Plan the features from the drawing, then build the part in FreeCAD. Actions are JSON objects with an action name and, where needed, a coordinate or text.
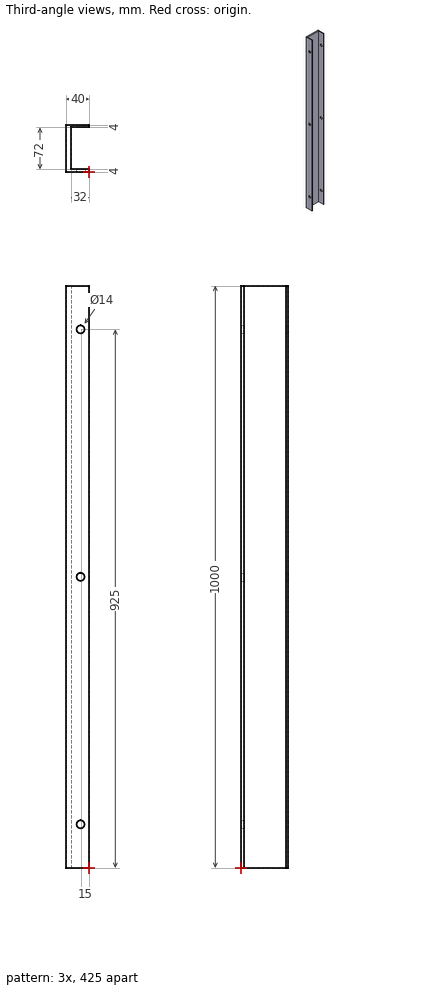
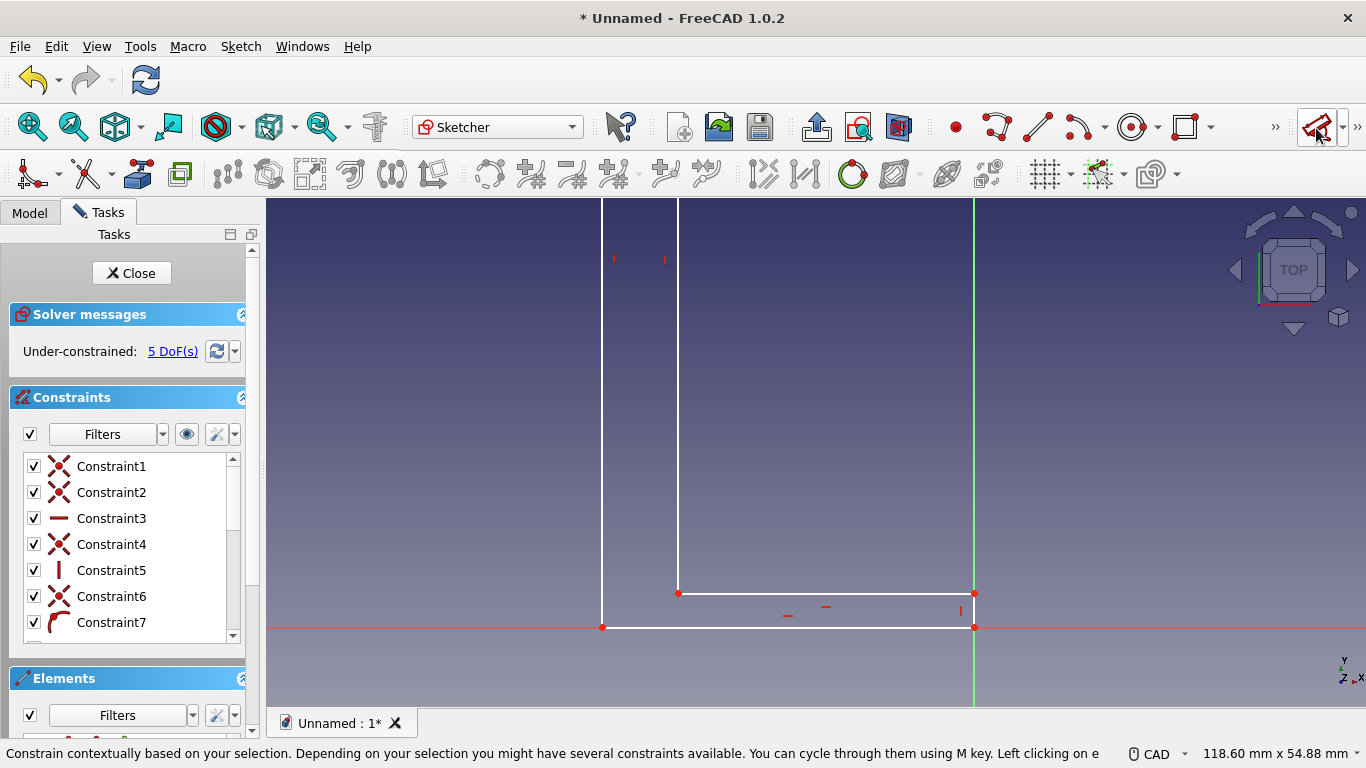
{"action": "scroll", "coordinate": [974, 618], "scroll_direction": "up", "scroll_amount": 2}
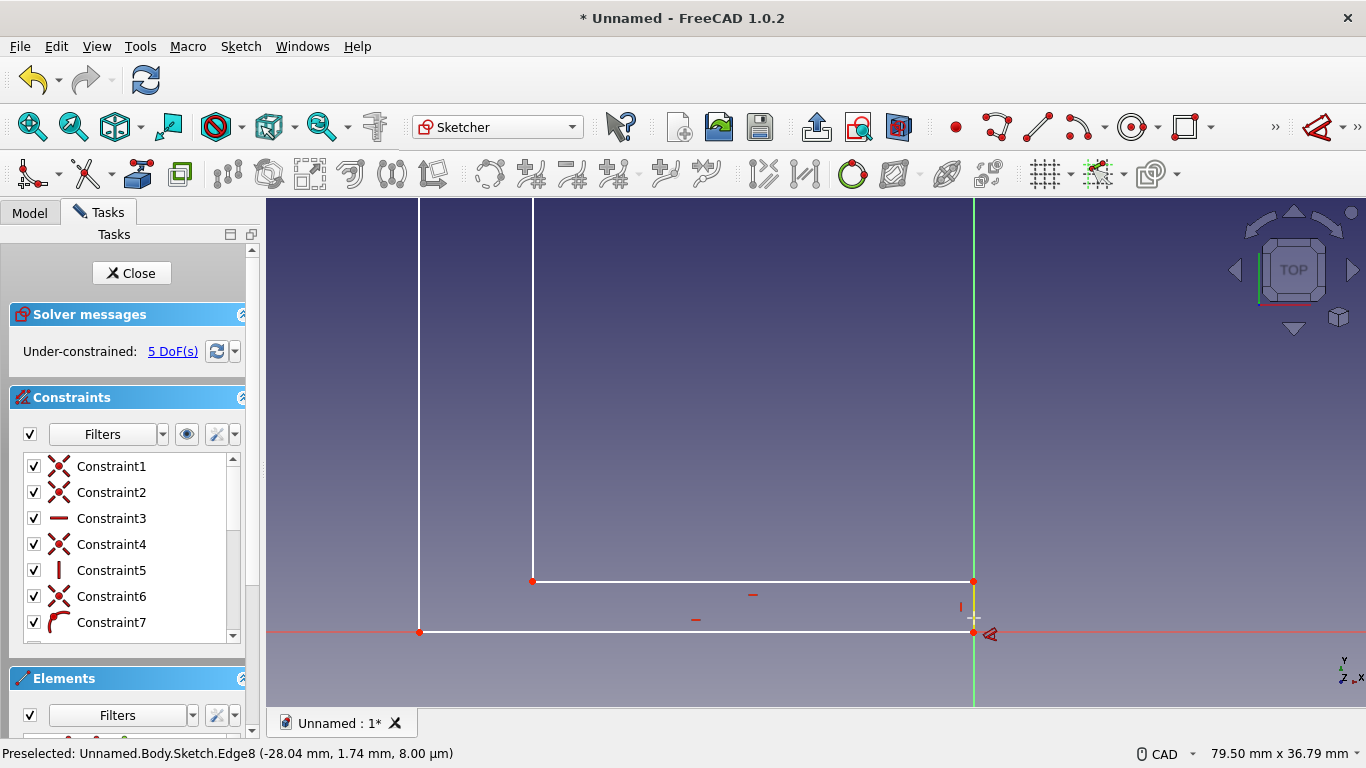
{"action": "left_click", "coordinate": [974, 617]}
{"action": "left_click", "coordinate": [1008, 607]}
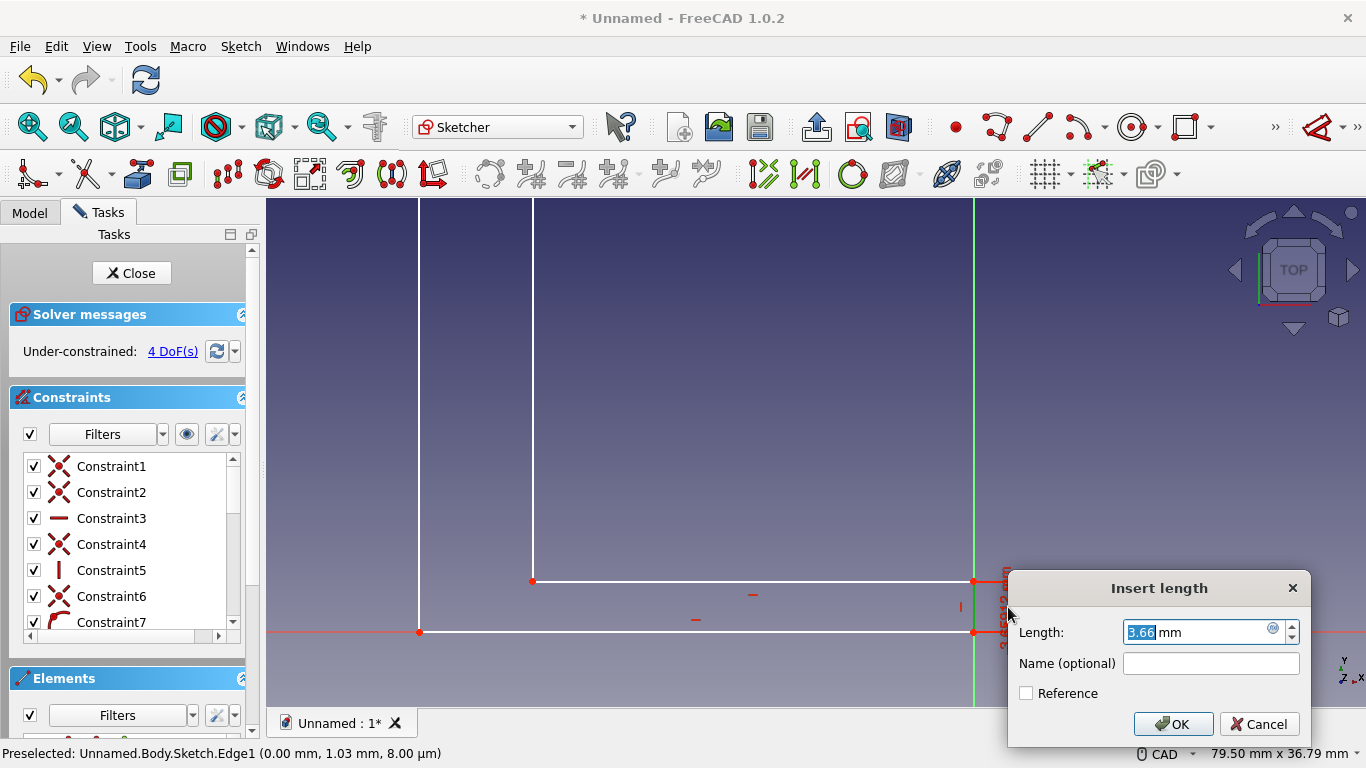
{"action": "type", "text": "4"}
{"action": "key", "text": "Return"}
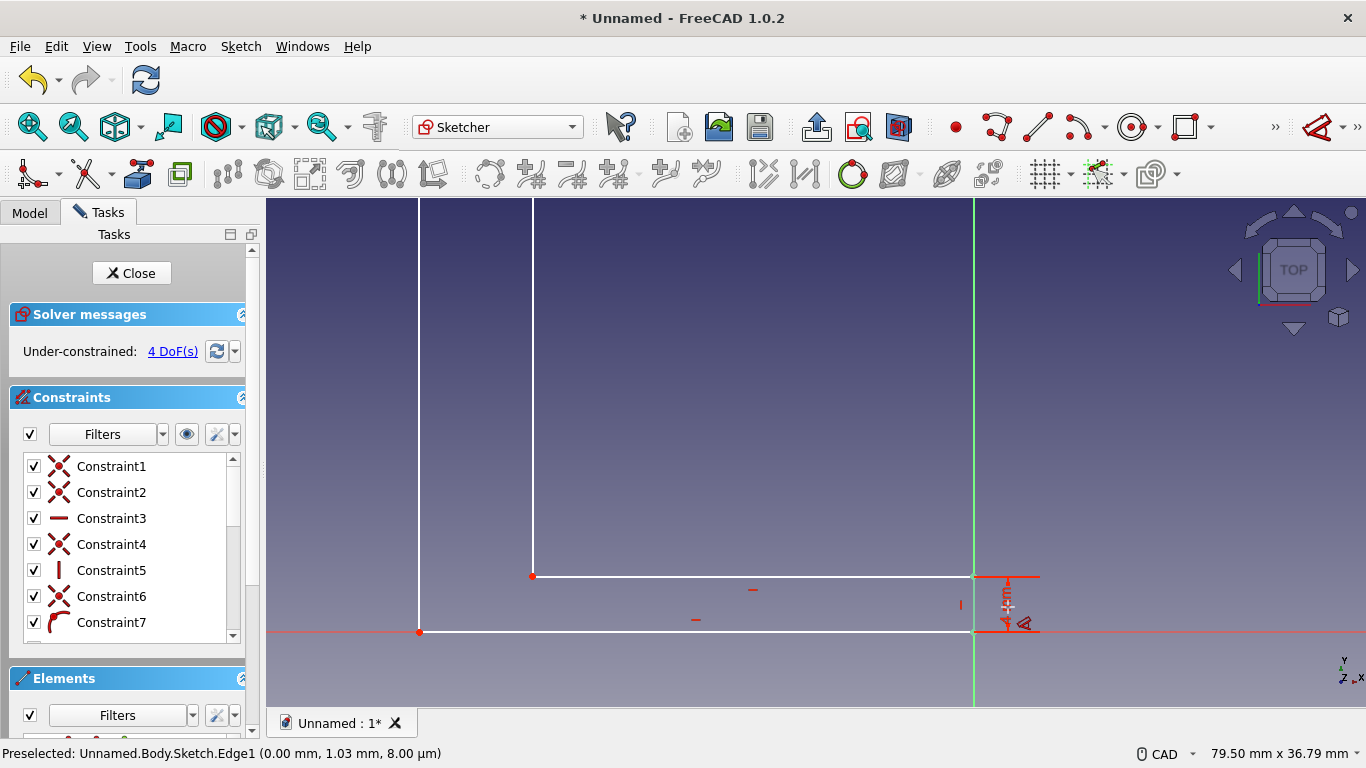
{"action": "scroll", "coordinate": [769, 614], "scroll_direction": "down", "scroll_amount": 6}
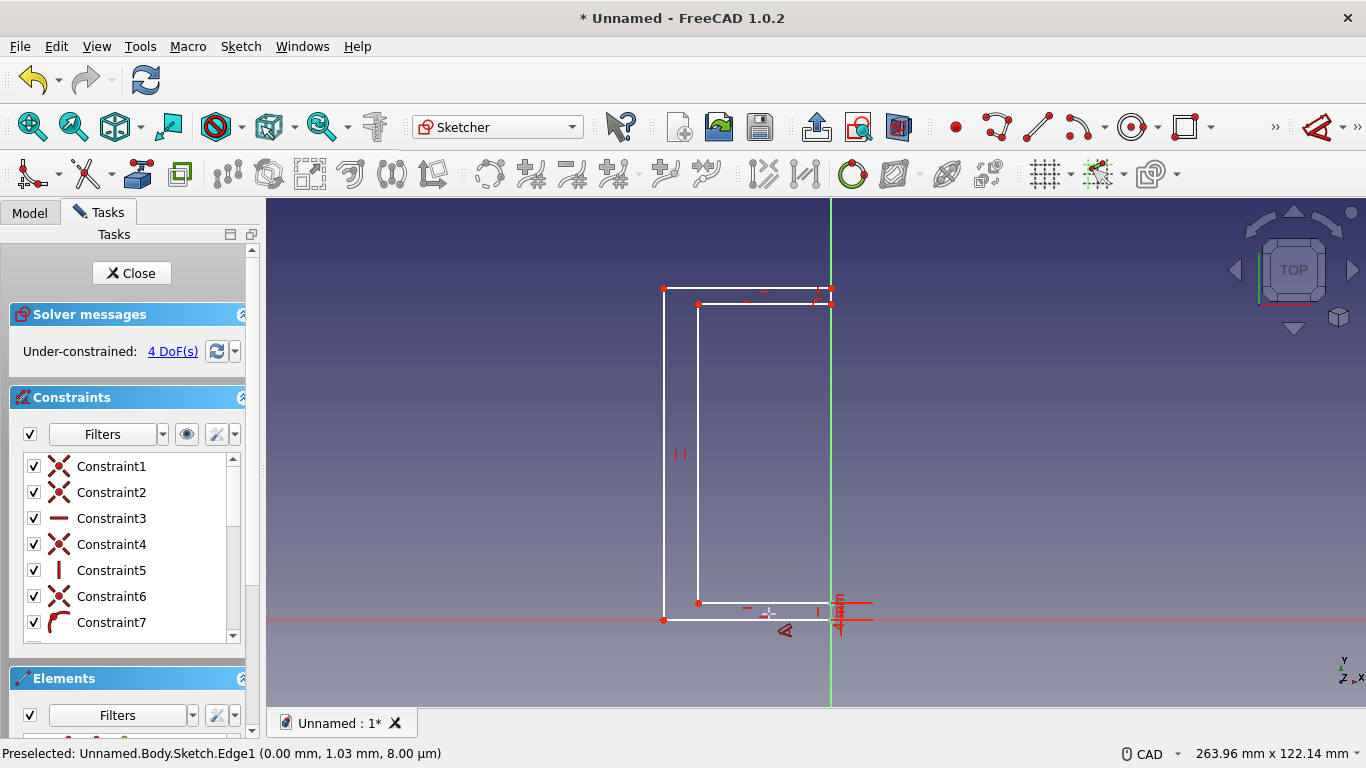
{"action": "scroll", "coordinate": [831, 300], "scroll_direction": "up", "scroll_amount": 6}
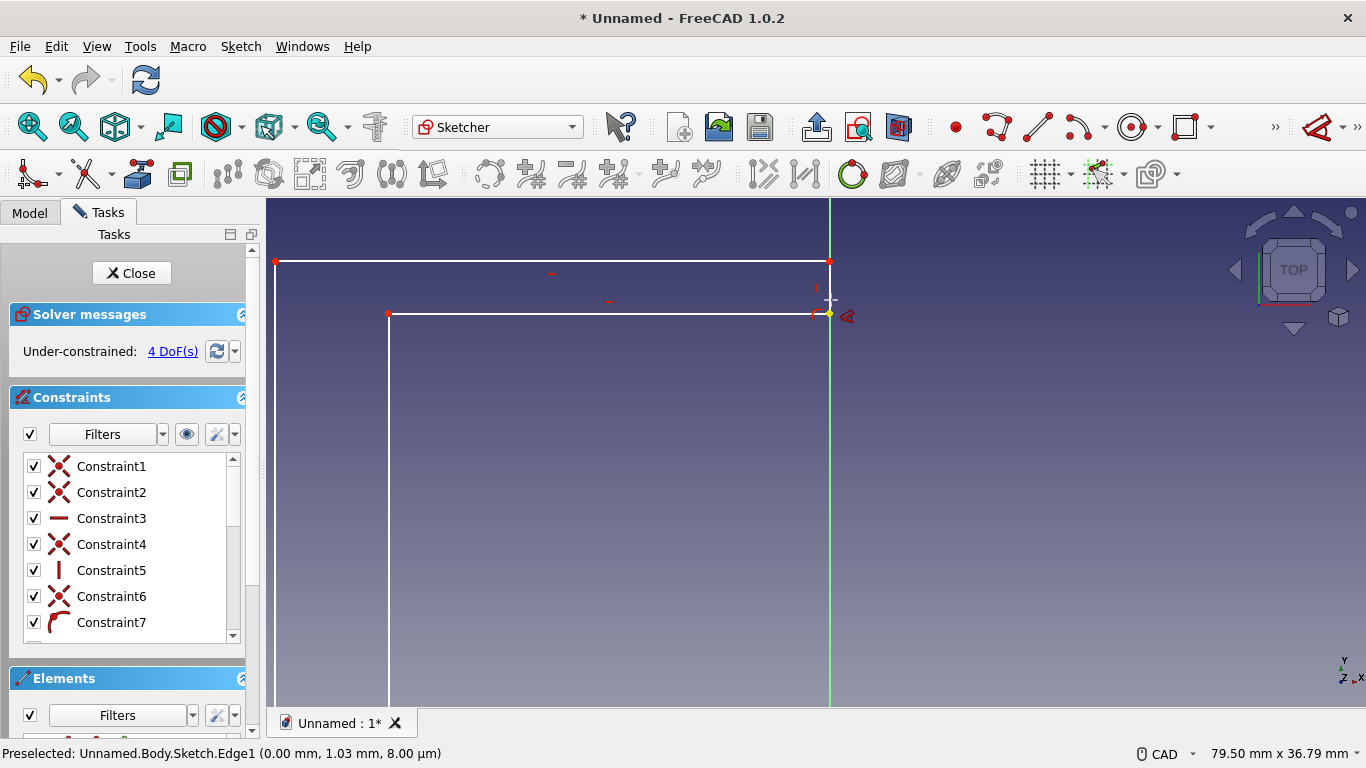
{"action": "left_click", "coordinate": [830, 298]}
{"action": "left_click", "coordinate": [864, 288]}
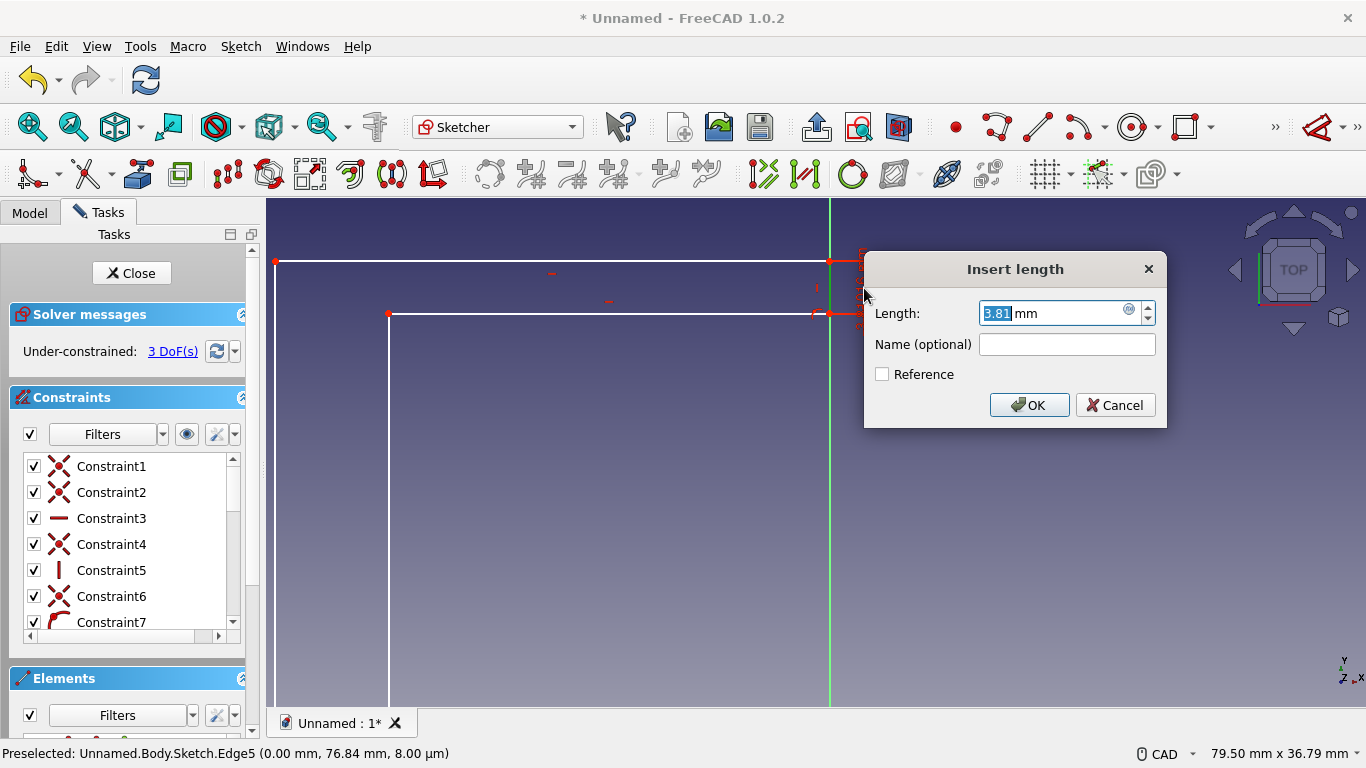
{"action": "type", "text": "4"}
{"action": "key", "text": "Return"}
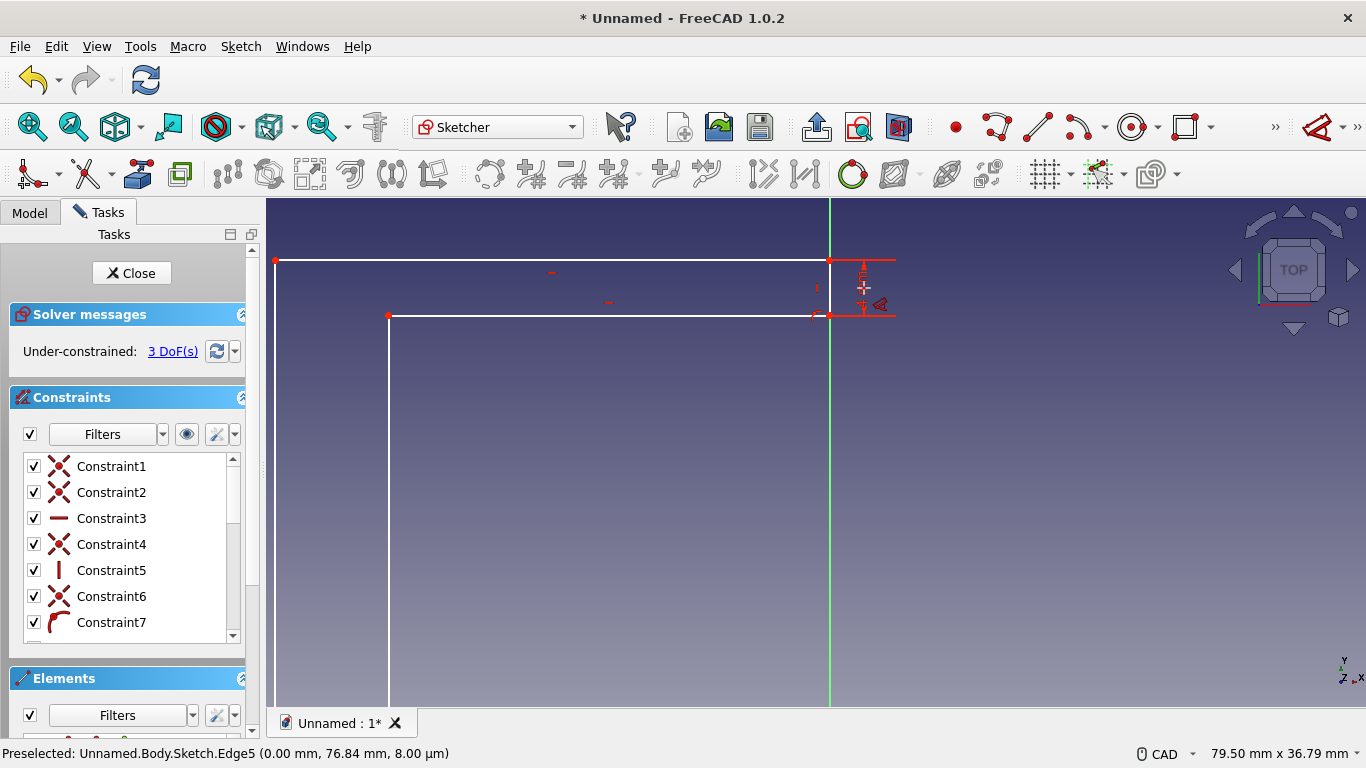
{"action": "scroll", "coordinate": [831, 299], "scroll_direction": "down", "scroll_amount": 6}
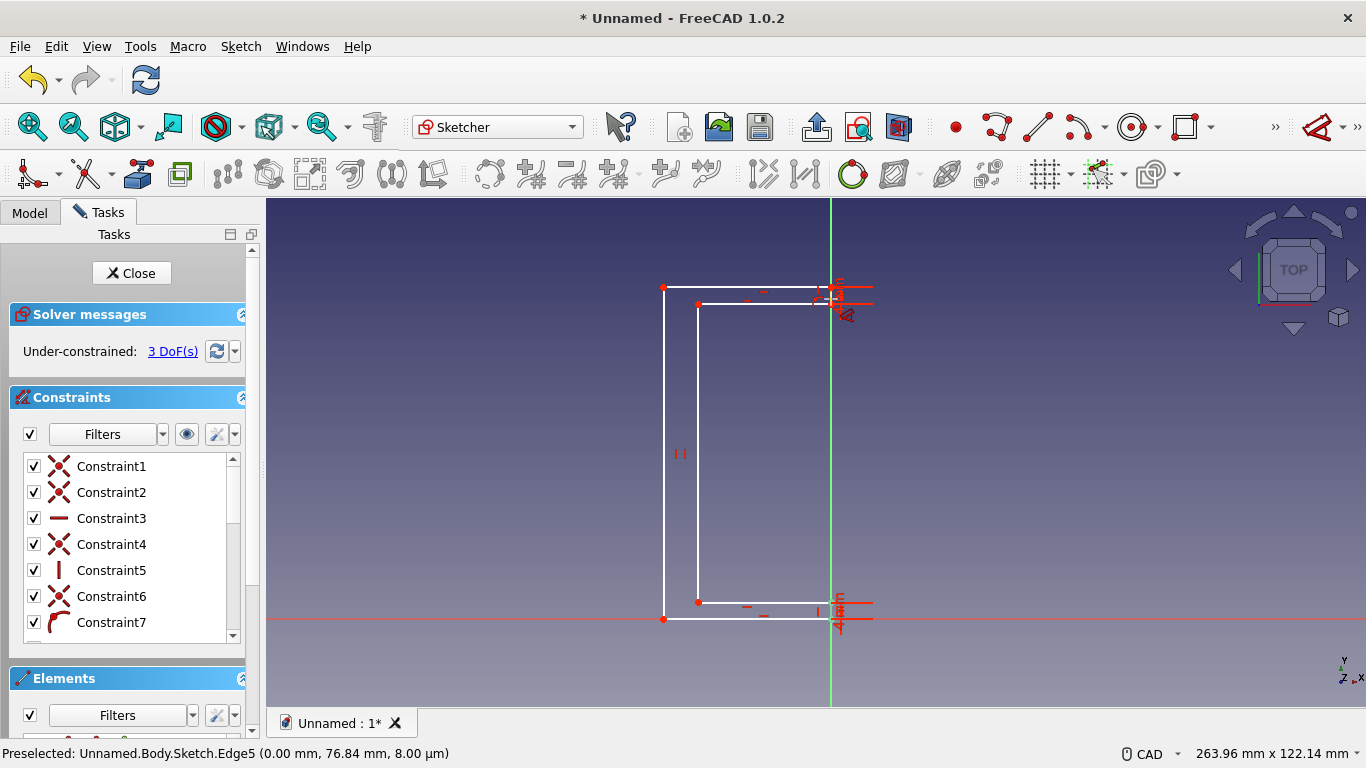
{"action": "left_click", "coordinate": [791, 603]}
{"action": "left_click", "coordinate": [765, 637]}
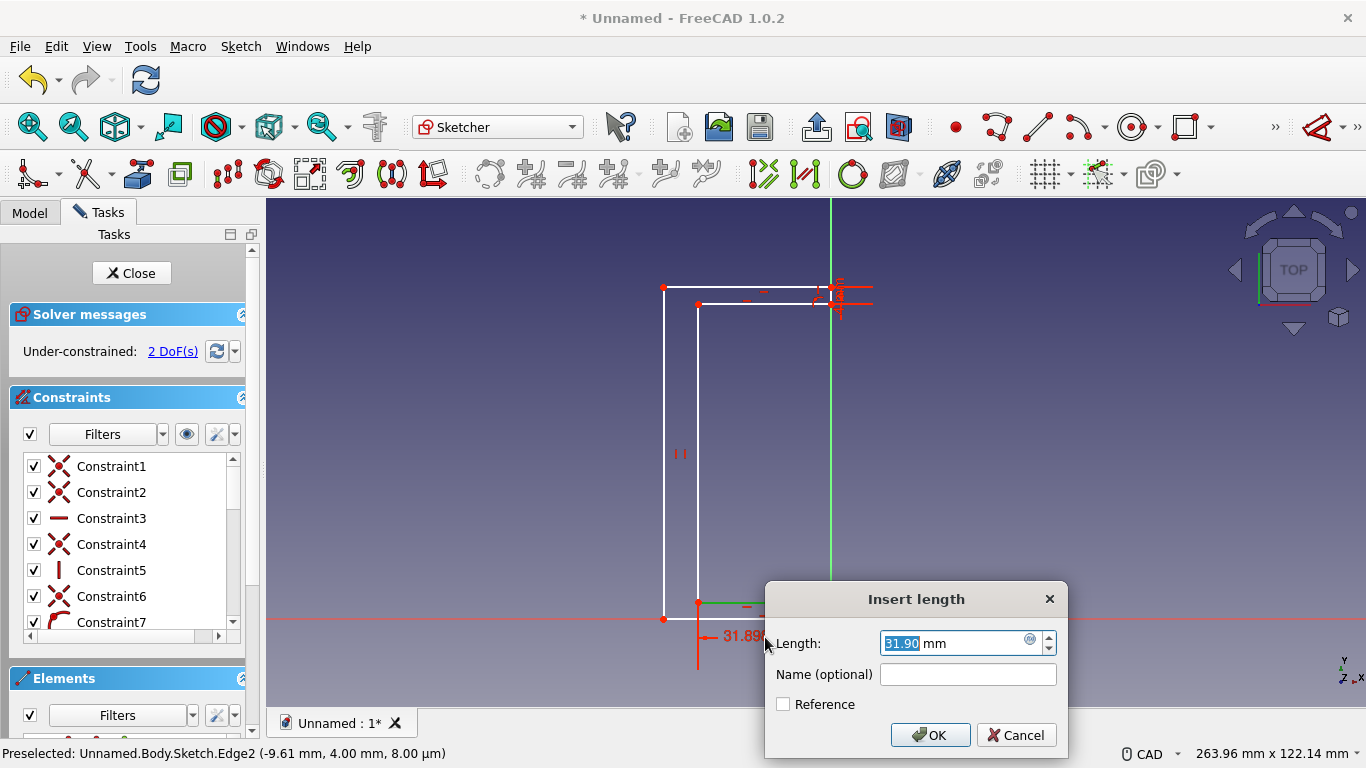
{"action": "type", "text": "32"}
{"action": "key", "text": "Return"}